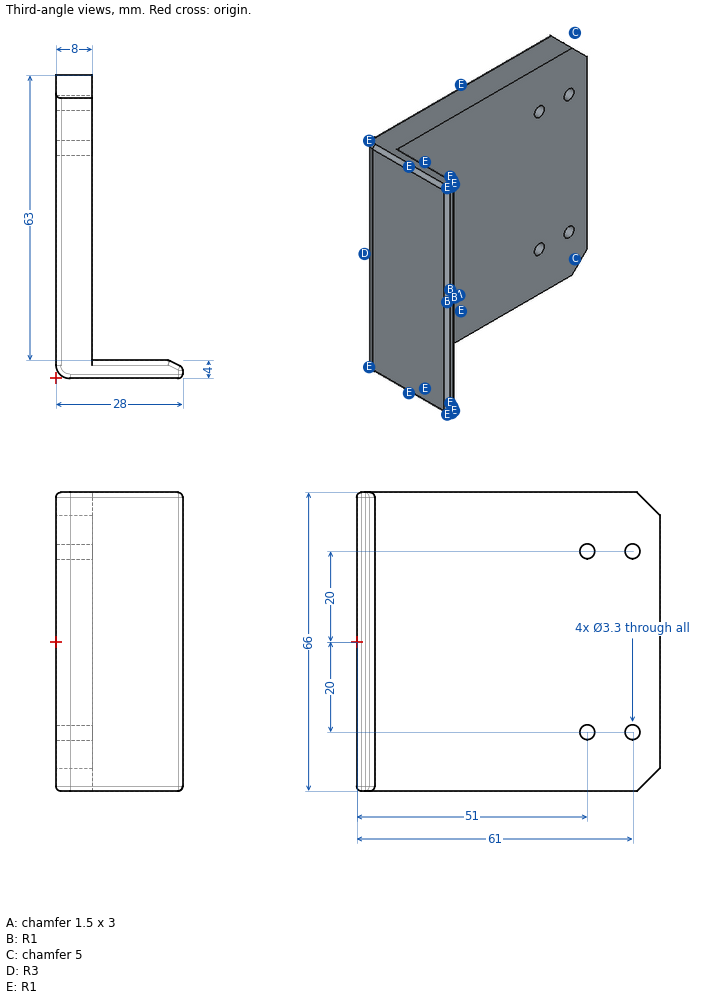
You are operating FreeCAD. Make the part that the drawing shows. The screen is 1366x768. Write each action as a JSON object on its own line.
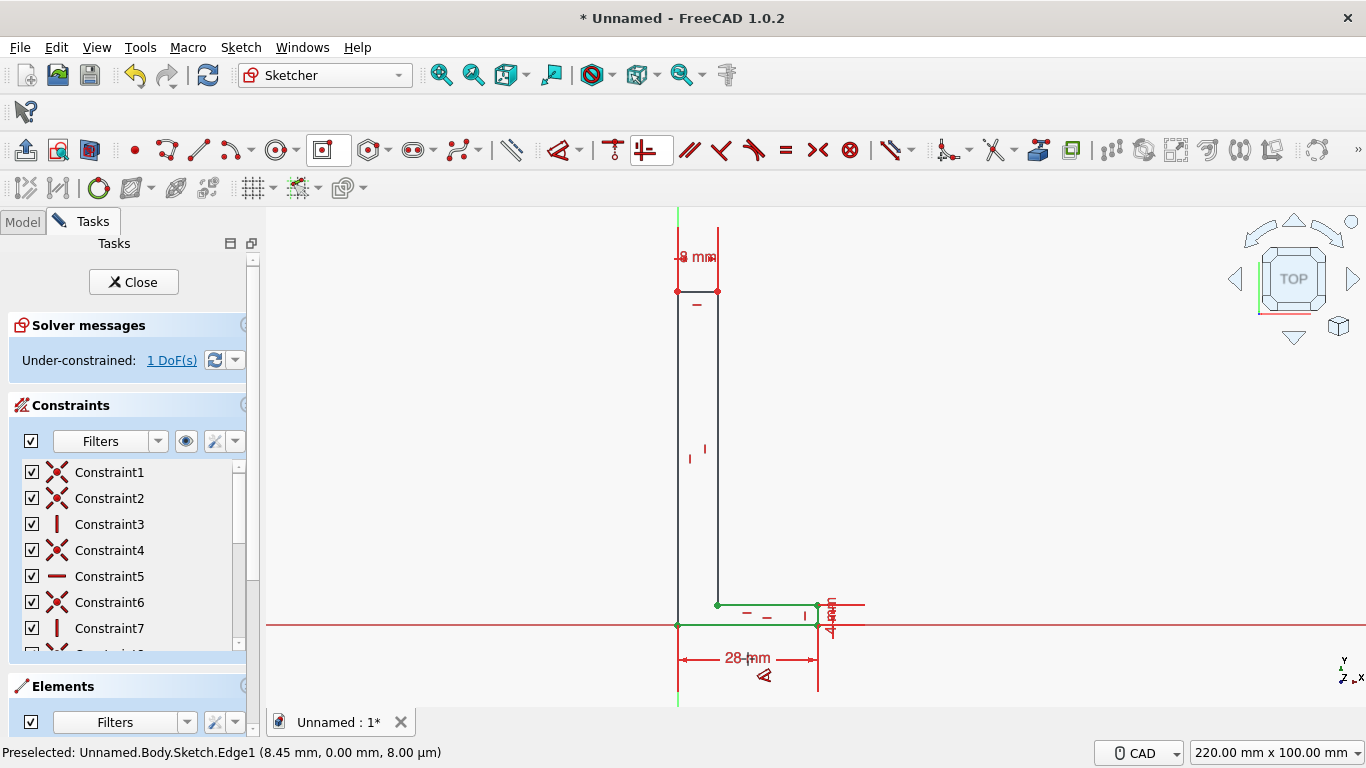
{"action": "left_click", "coordinate": [718, 511]}
{"action": "left_click", "coordinate": [752, 448]}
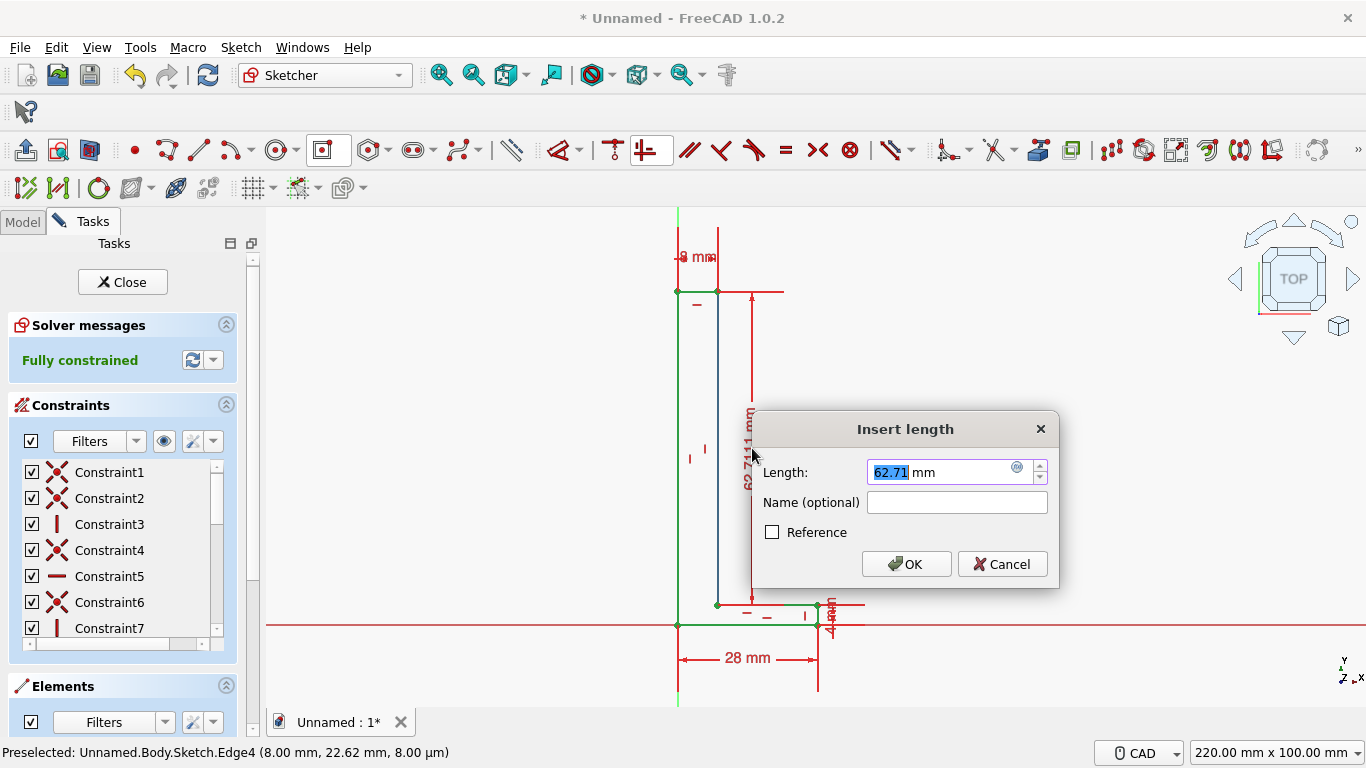
{"action": "type", "text": "63"}
{"action": "key", "text": "Return"}
{"action": "key", "text": "Escape"}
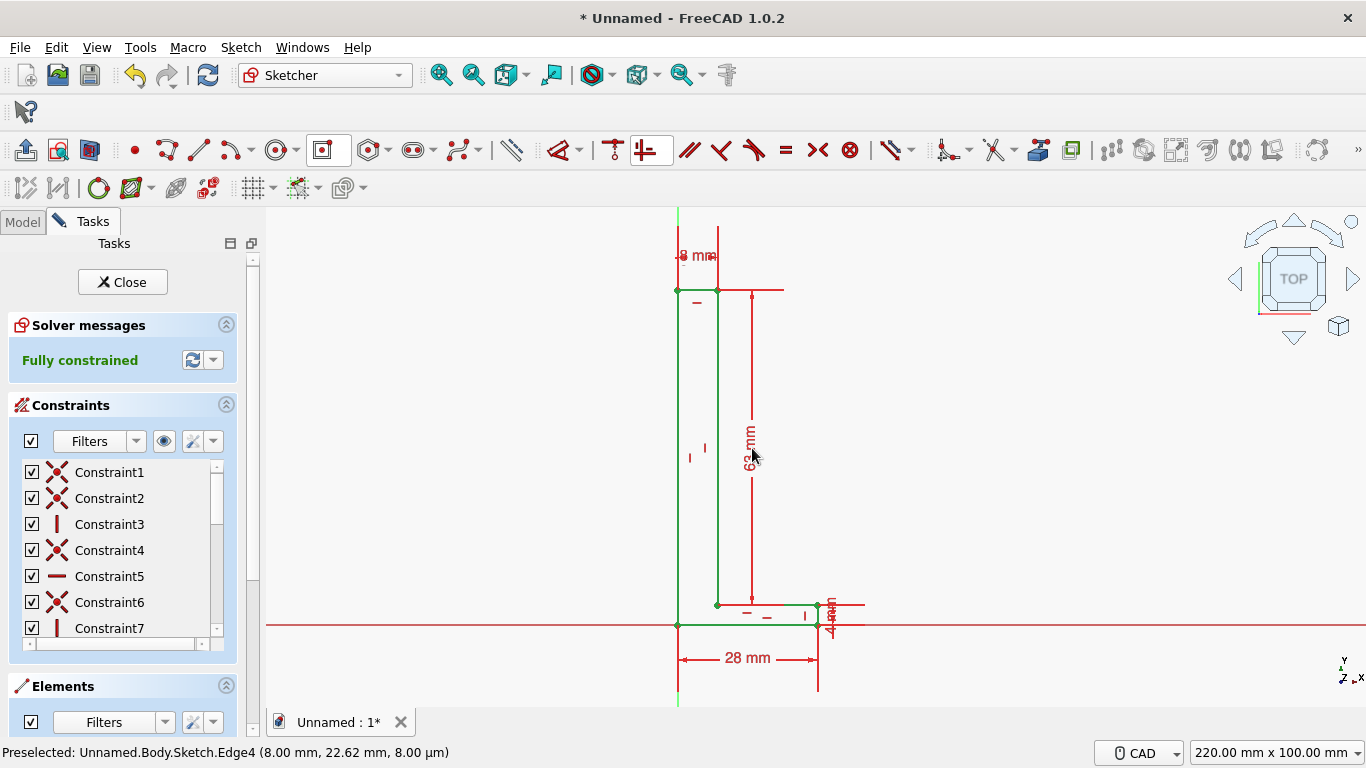
{"action": "left_click", "coordinate": [123, 282]}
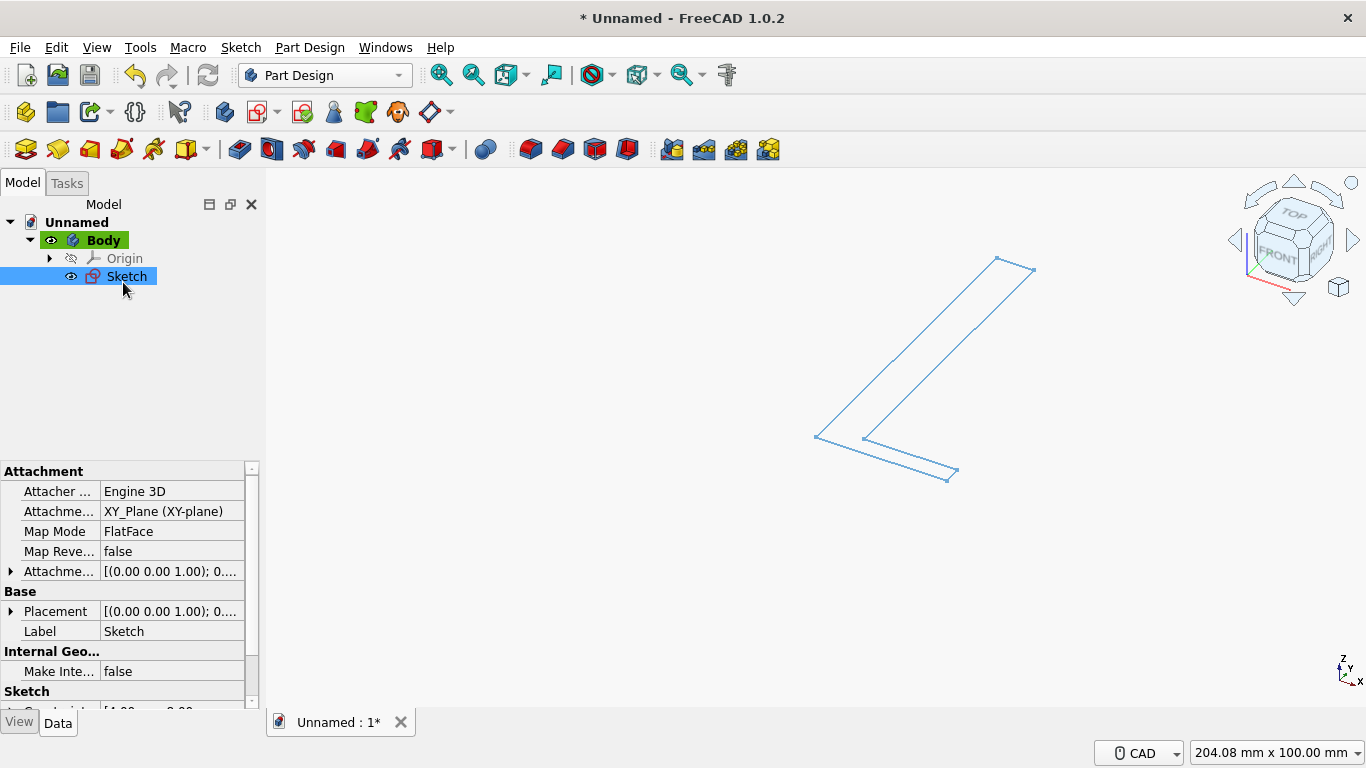
{"action": "left_click", "coordinate": [26, 150]}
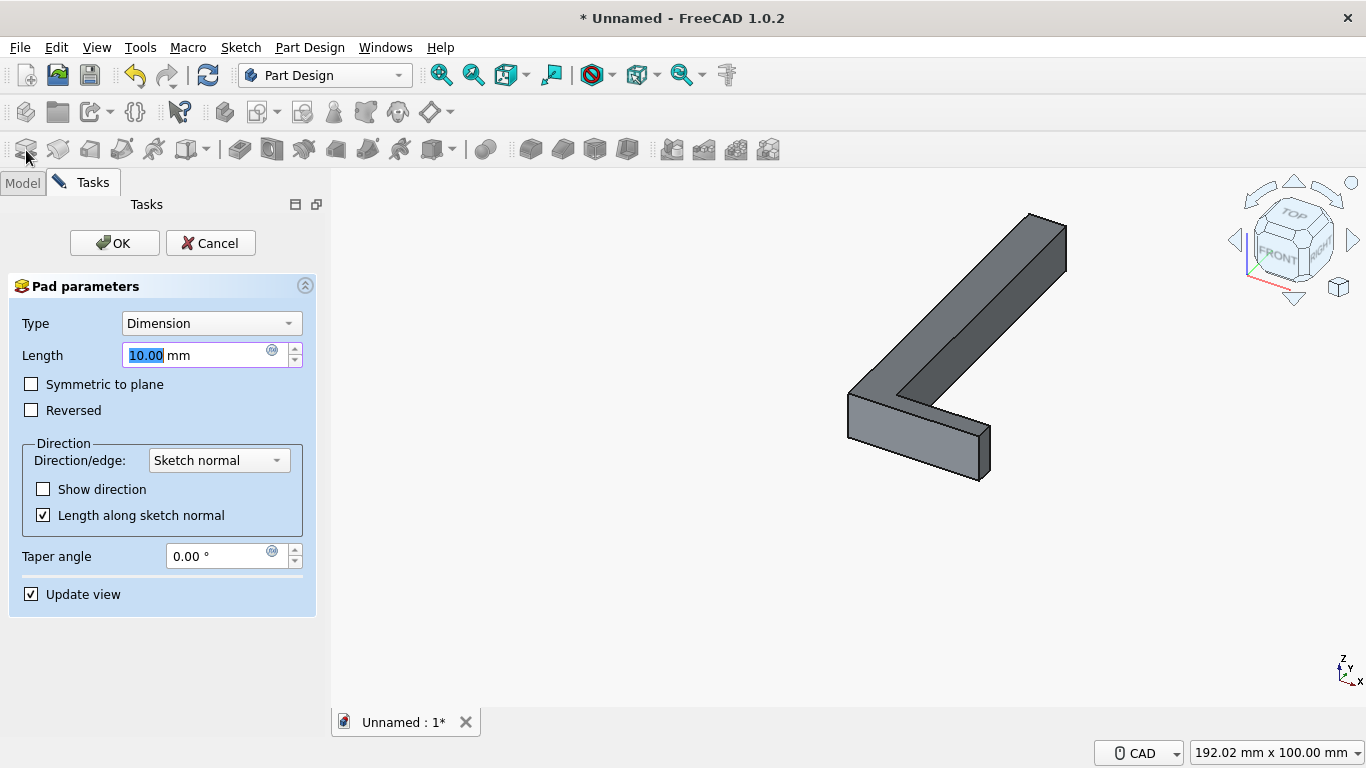
{"action": "type", "text": "66"}
{"action": "key", "text": "Tab"}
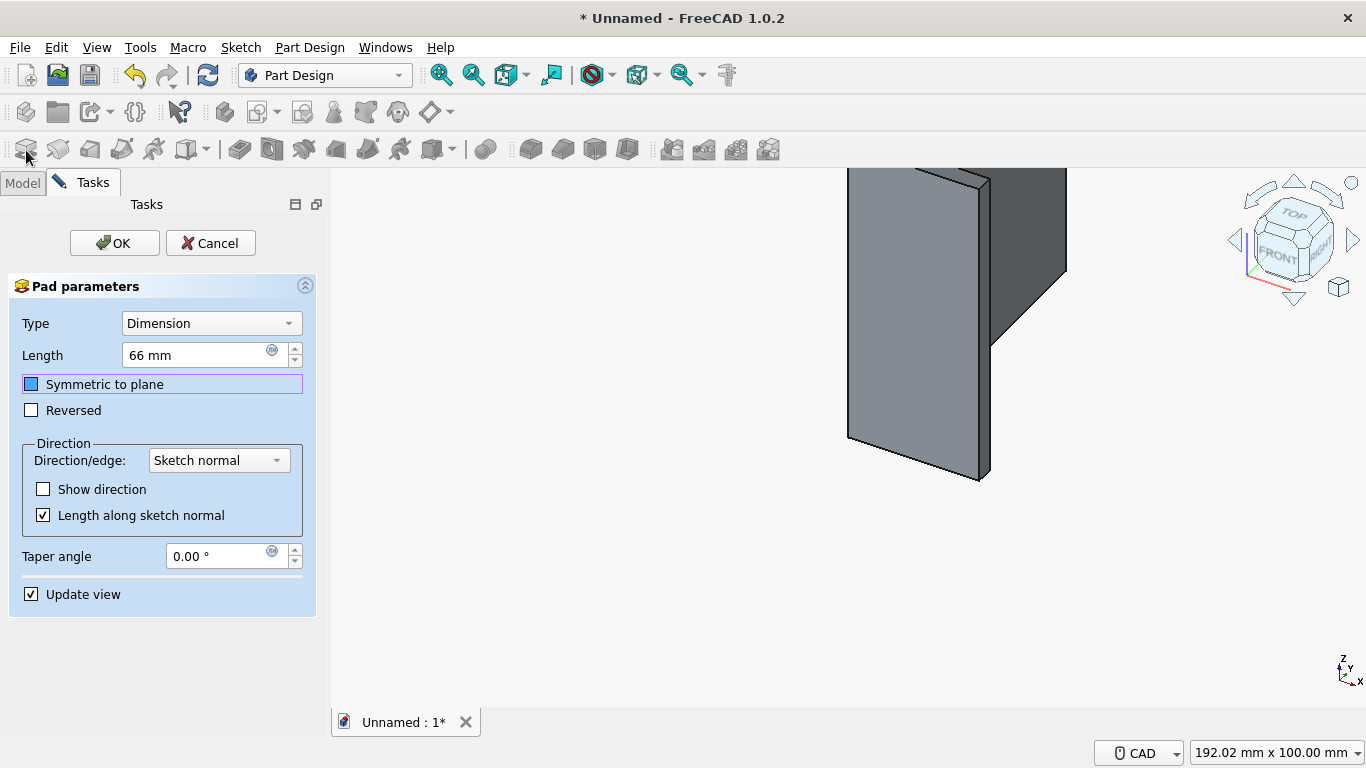
{"action": "left_click", "coordinate": [30, 384]}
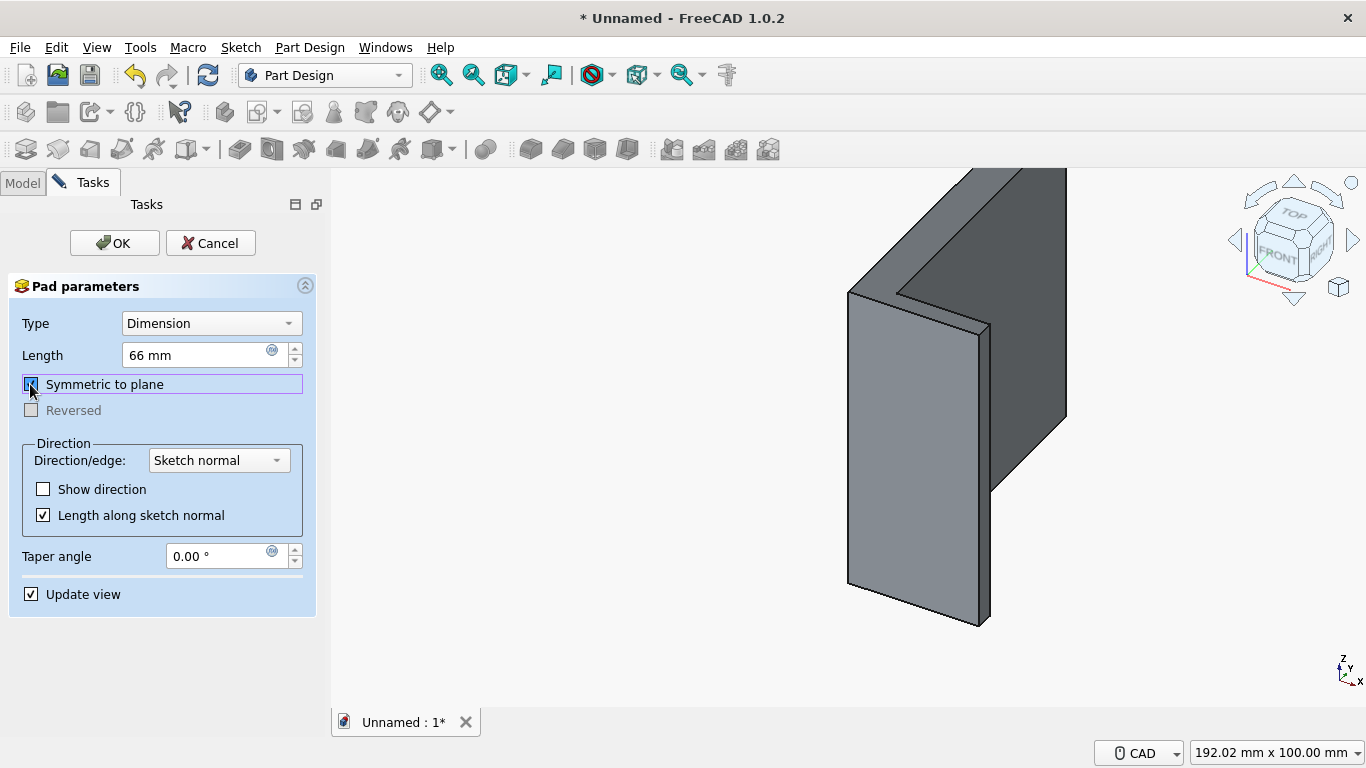
{"action": "left_click", "coordinate": [115, 243]}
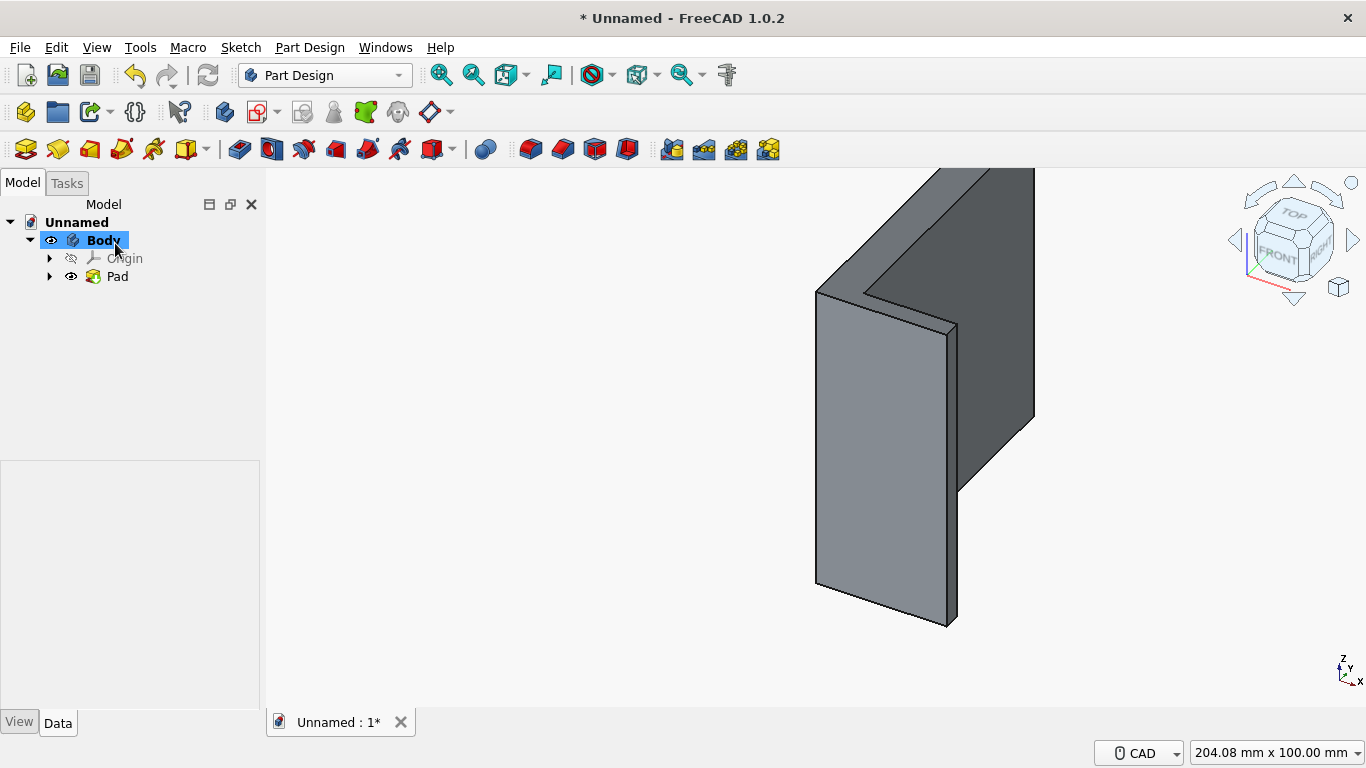
{"action": "left_click", "coordinate": [442, 76]}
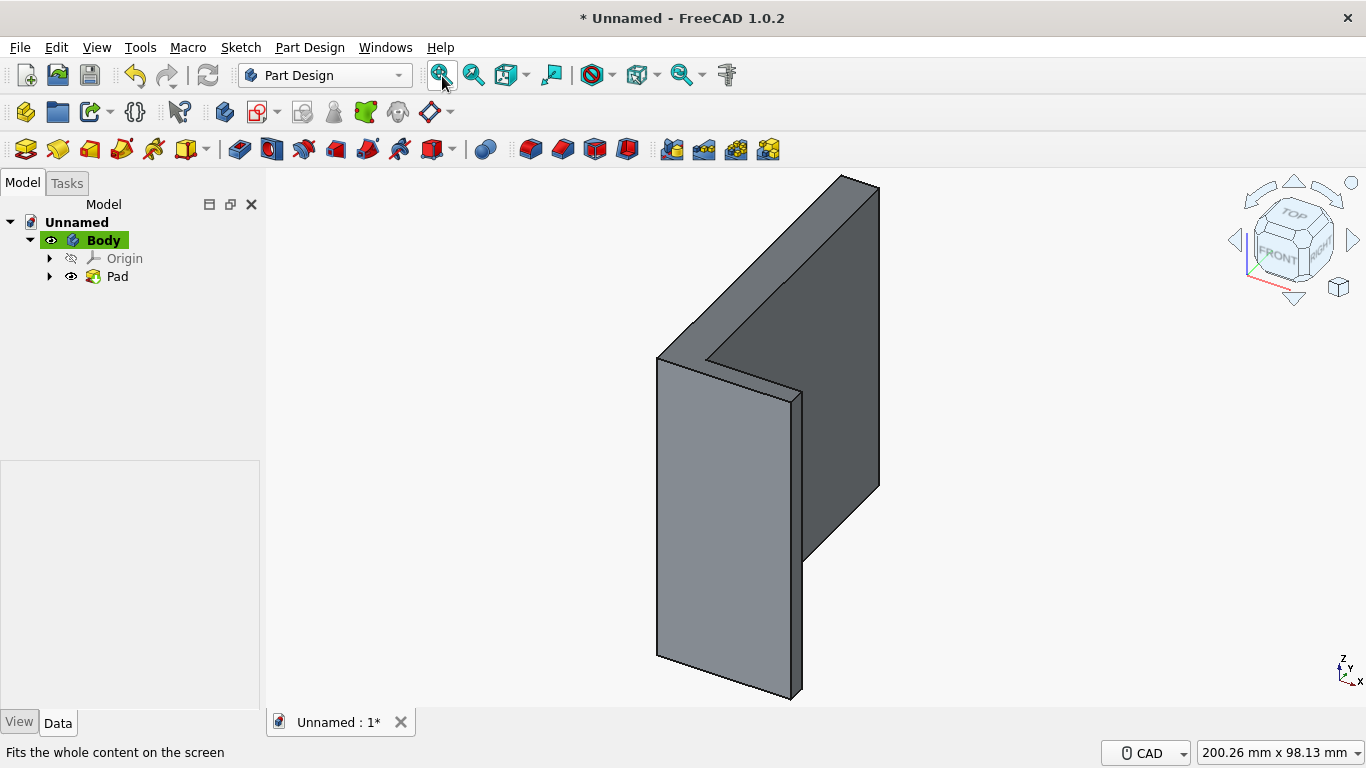
{"action": "key", "text": "0"}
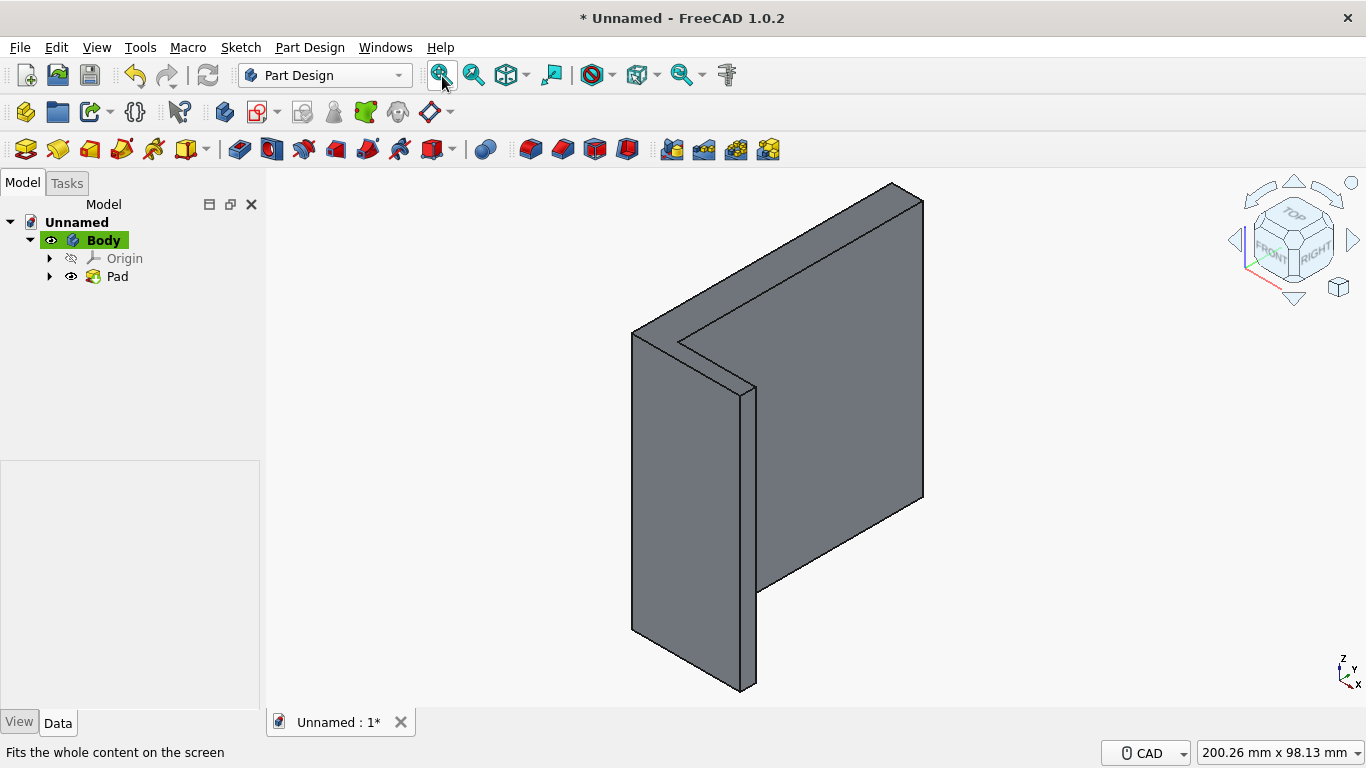
{"action": "key", "text": "2"}